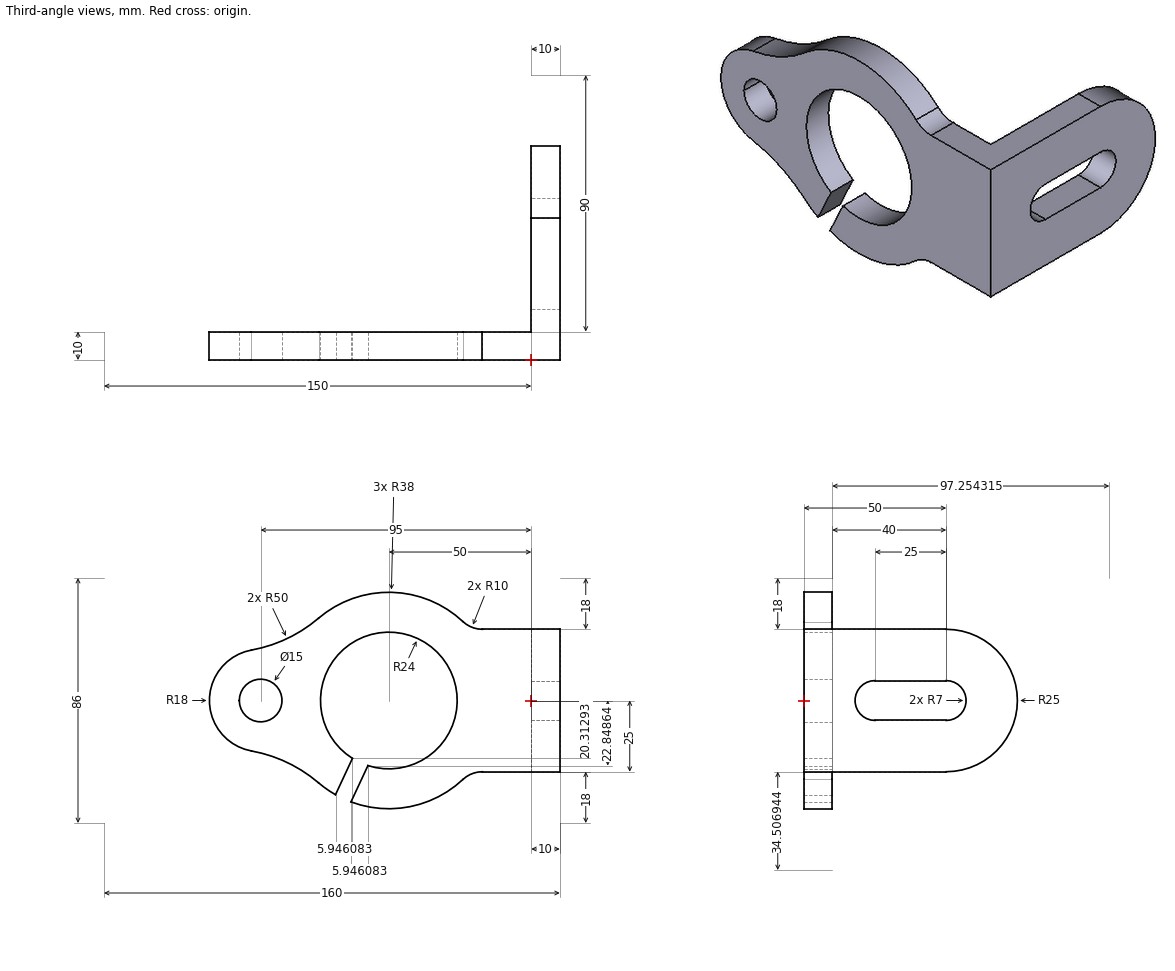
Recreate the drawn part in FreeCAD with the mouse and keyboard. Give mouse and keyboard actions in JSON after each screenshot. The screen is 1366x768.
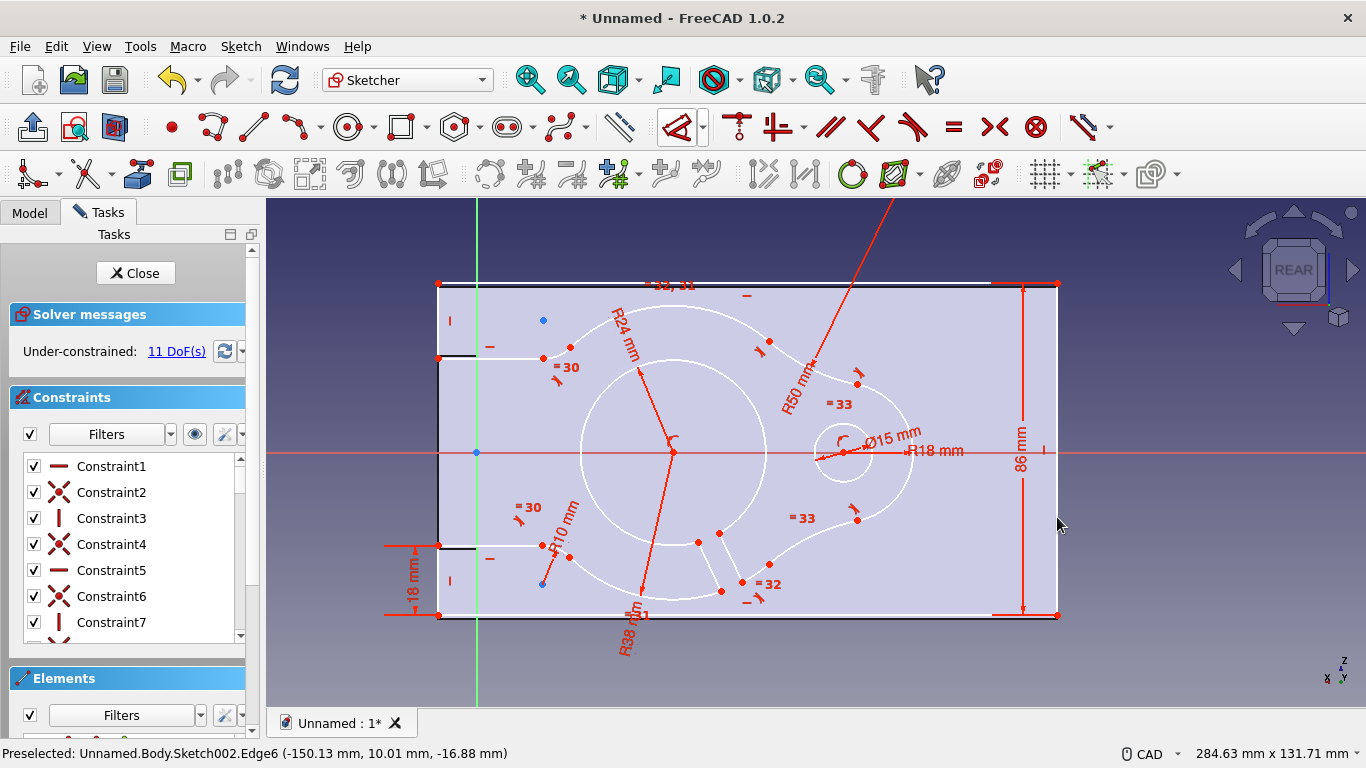
{"action": "left_click", "coordinate": [438, 306]}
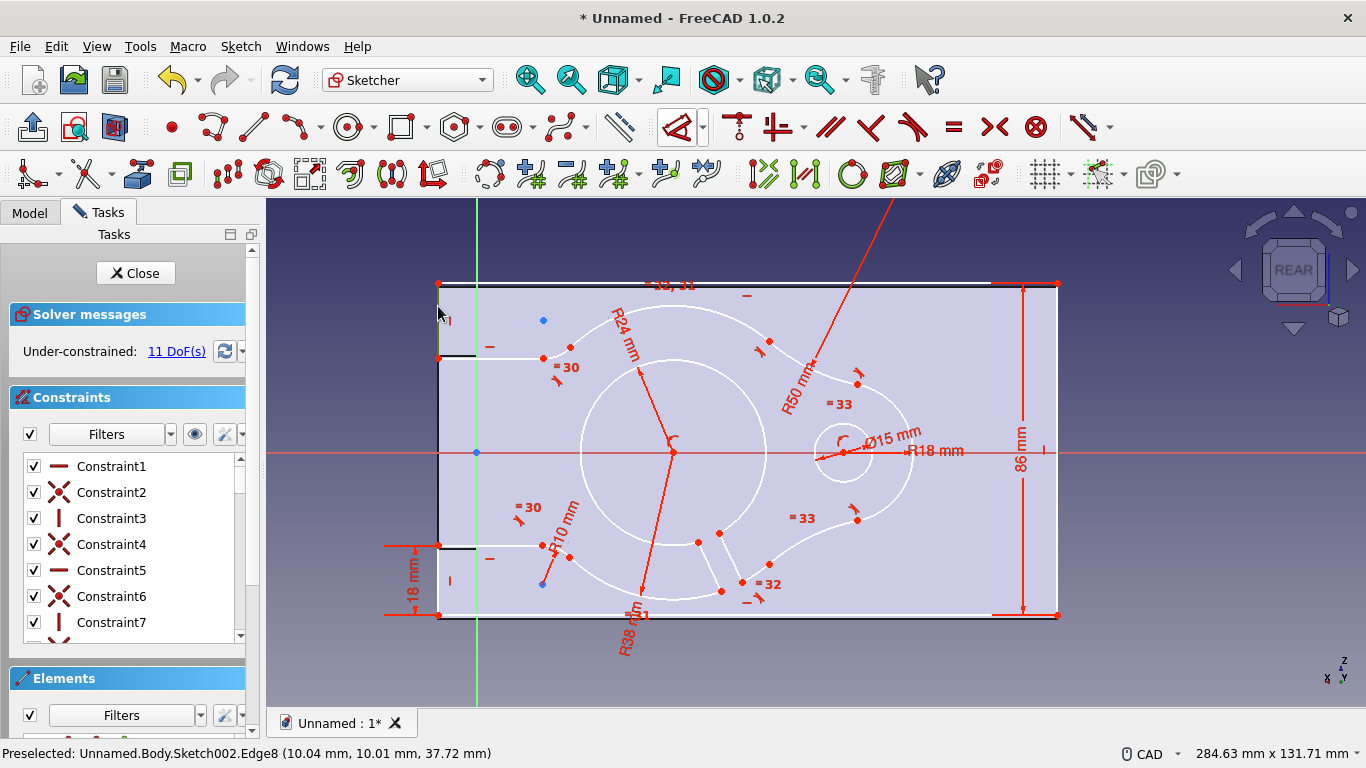
{"action": "left_click", "coordinate": [702, 128]}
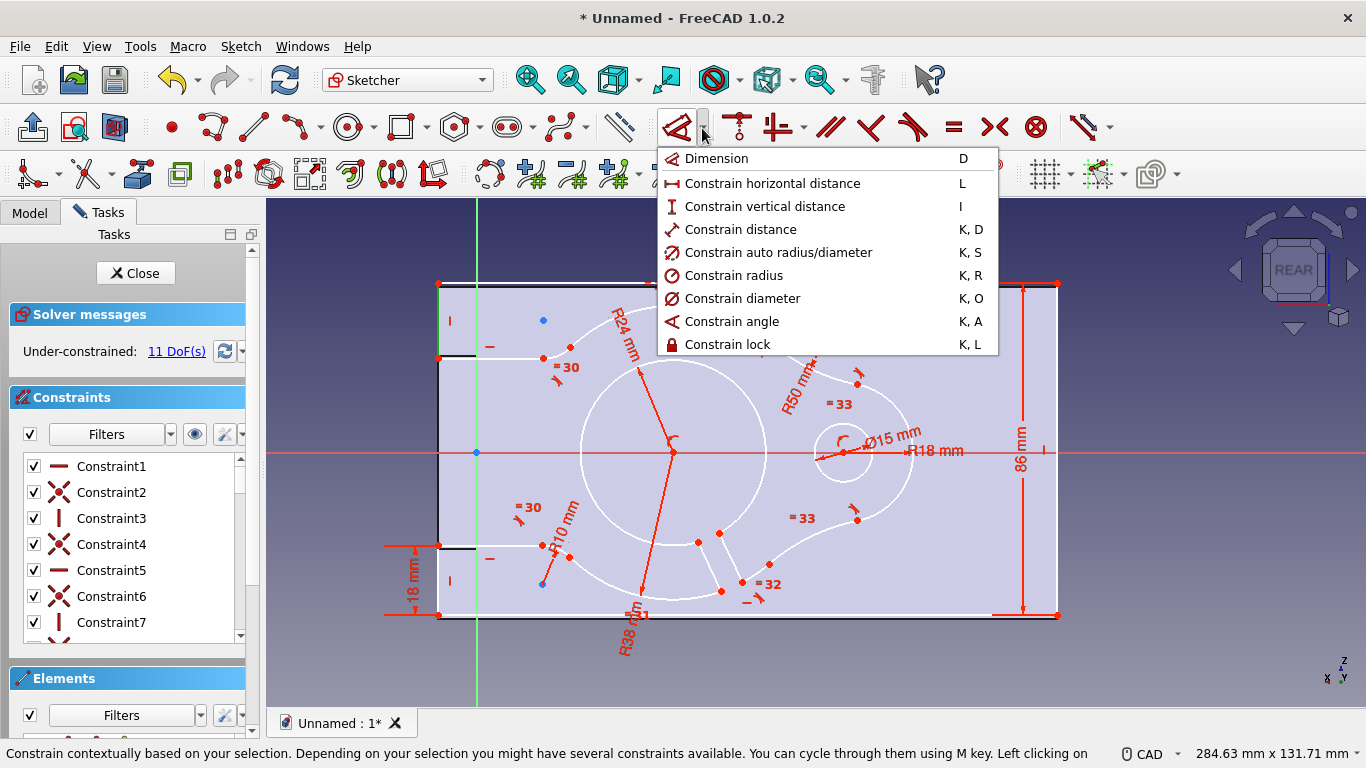
{"action": "left_click", "coordinate": [828, 206]}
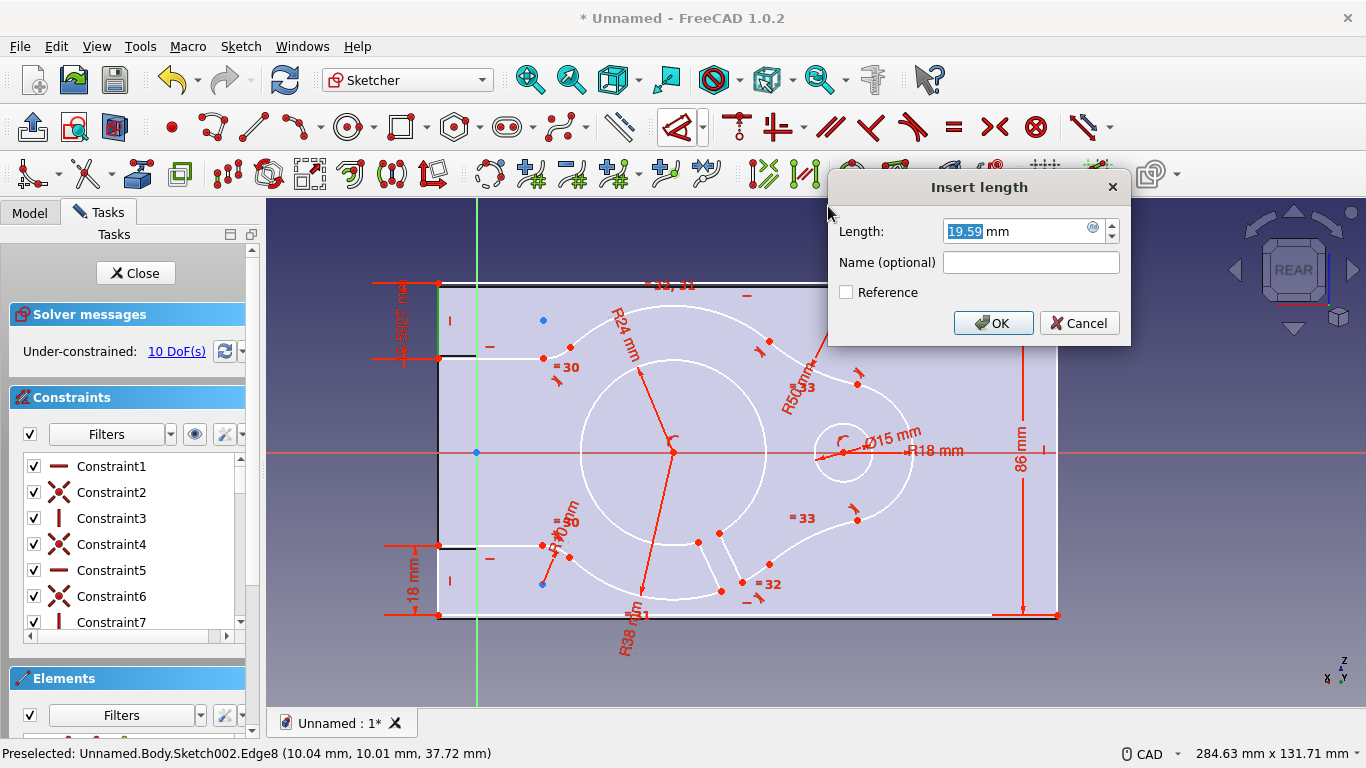
{"action": "type", "text": "18"}
{"action": "key", "text": "Return"}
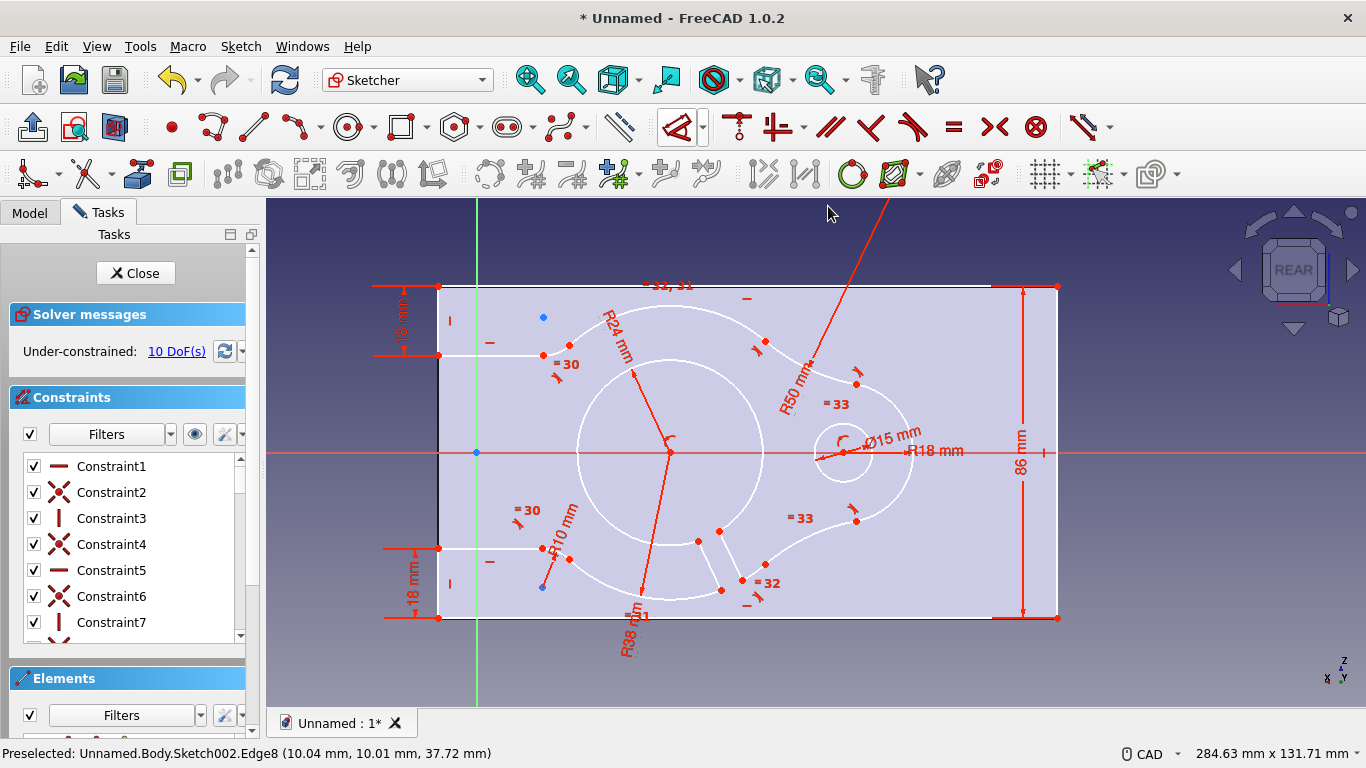
{"action": "left_click", "coordinate": [844, 453]}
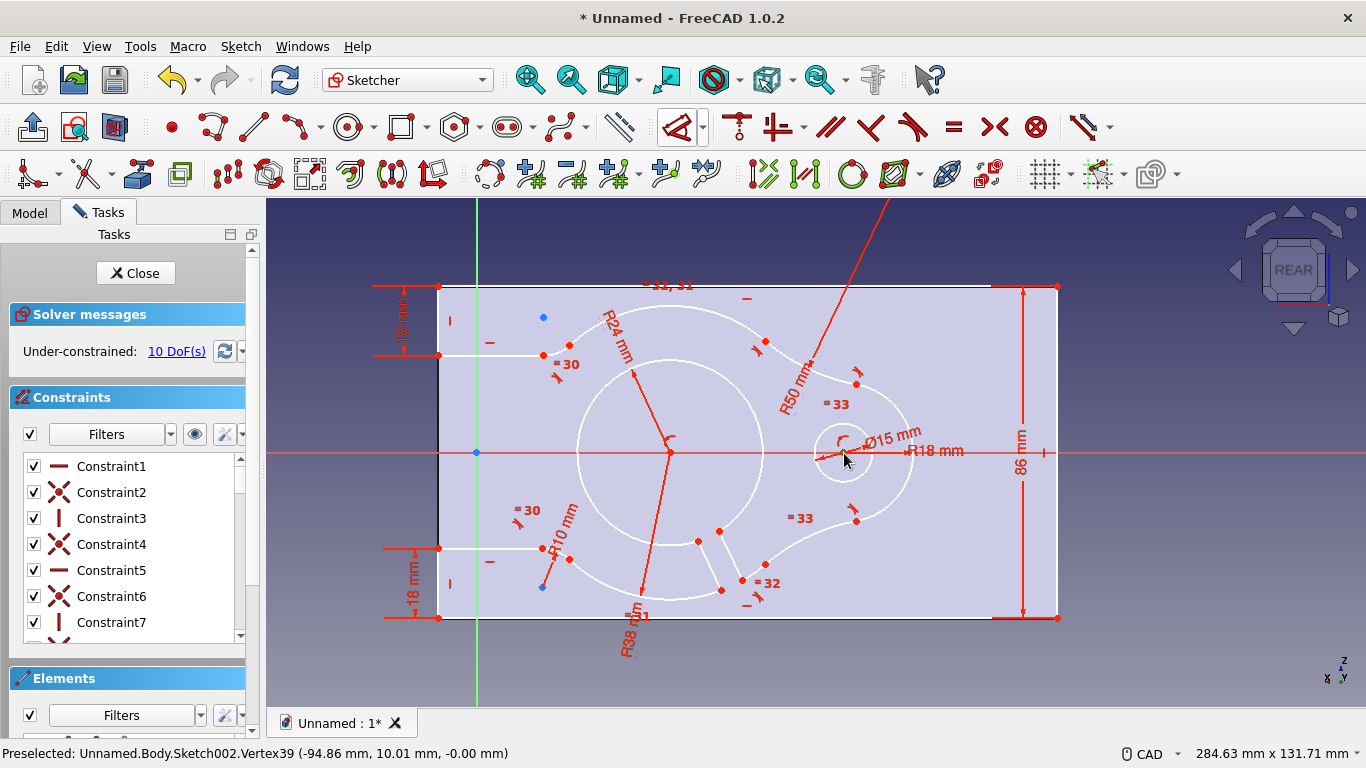
{"action": "left_click", "coordinate": [702, 128]}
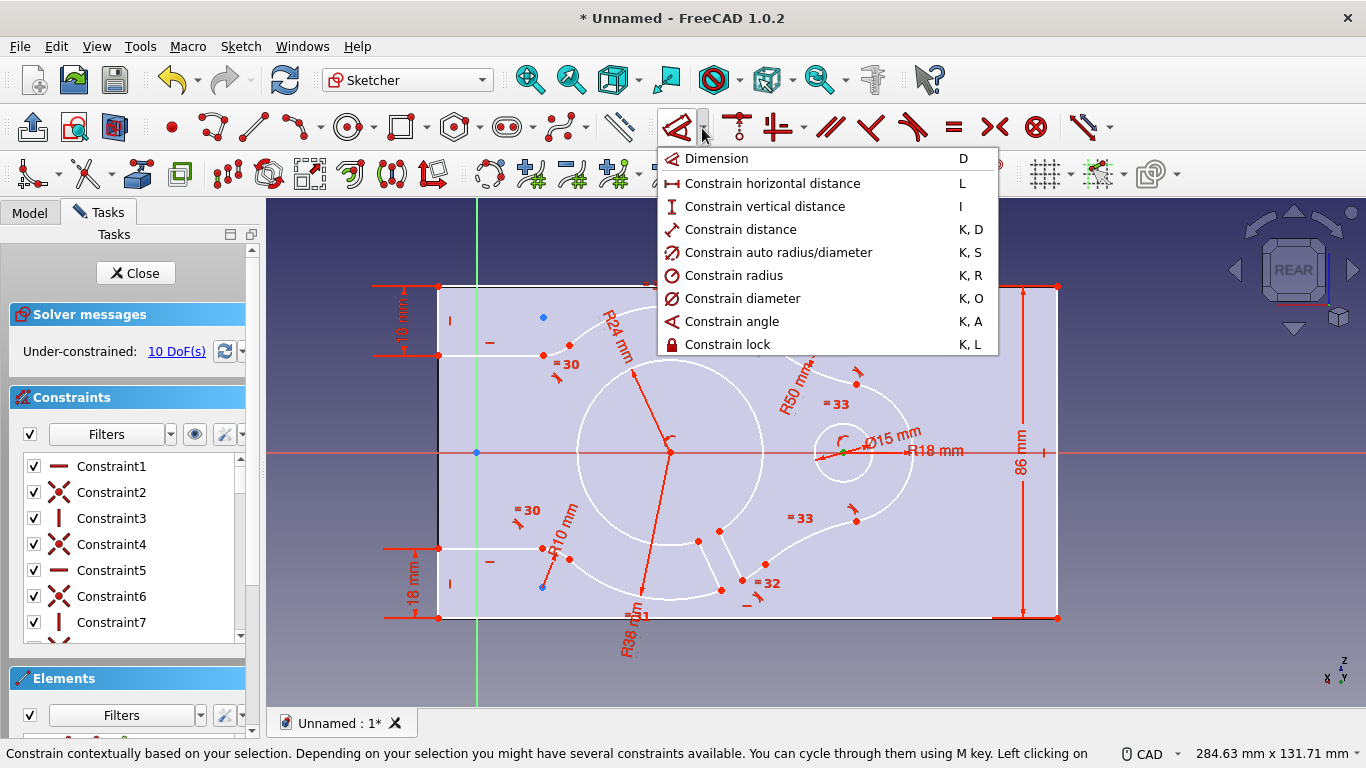
{"action": "left_click", "coordinate": [828, 184]}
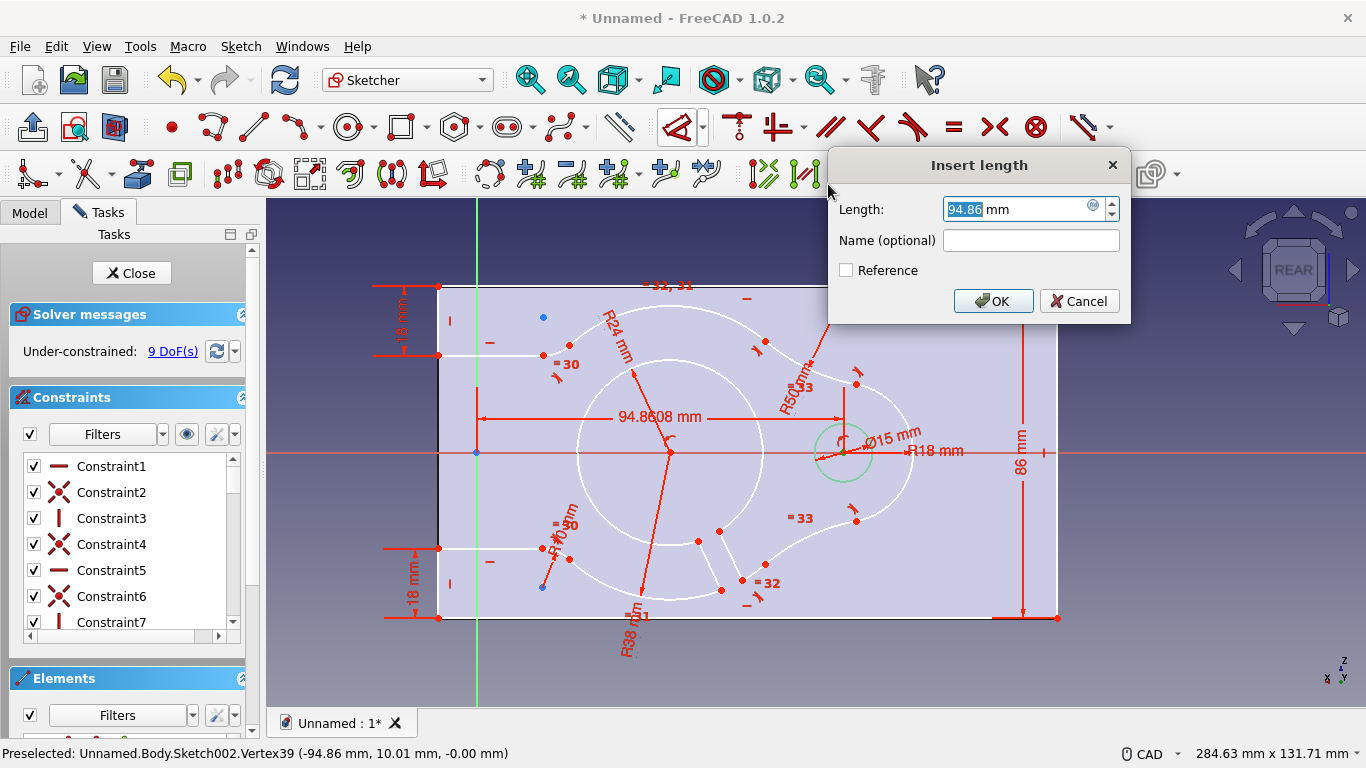
{"action": "type", "text": "95"}
{"action": "key", "text": "Return"}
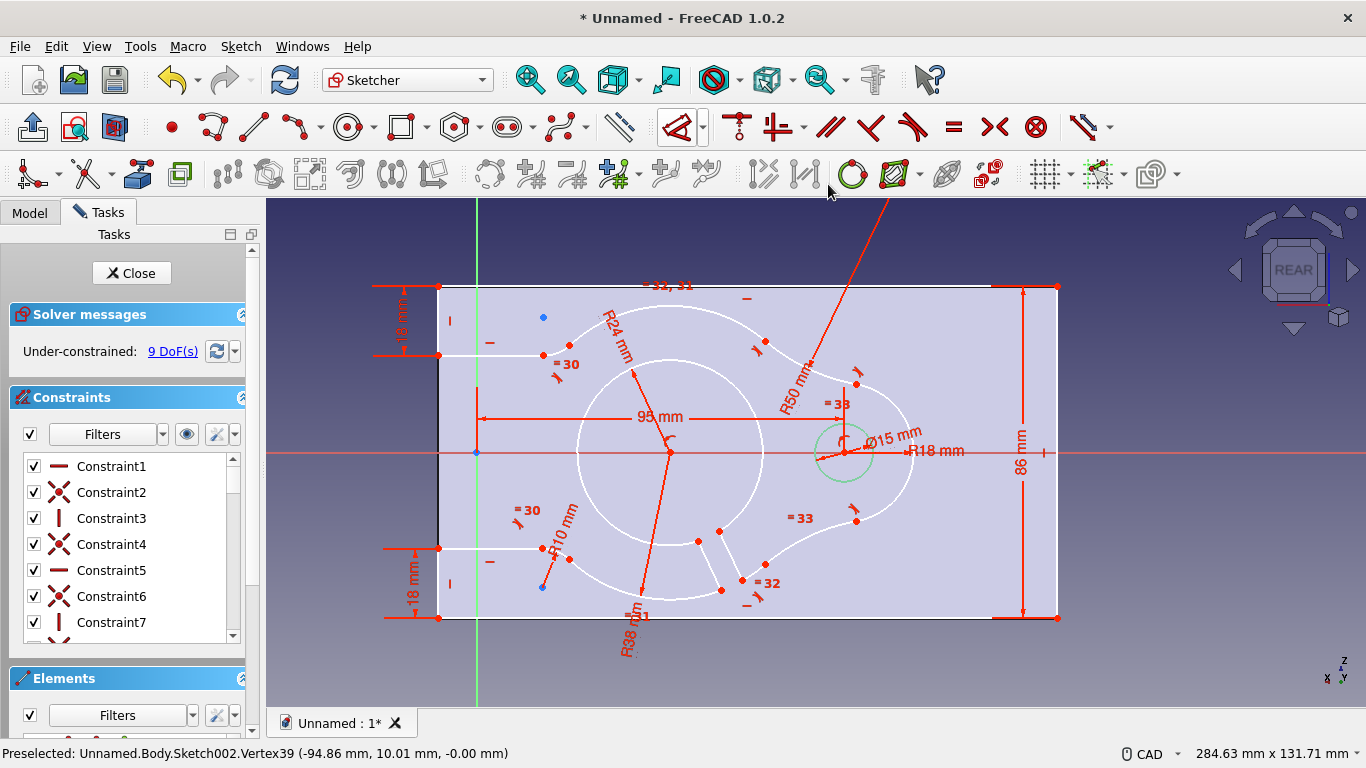
{"action": "left_click", "coordinate": [871, 618]}